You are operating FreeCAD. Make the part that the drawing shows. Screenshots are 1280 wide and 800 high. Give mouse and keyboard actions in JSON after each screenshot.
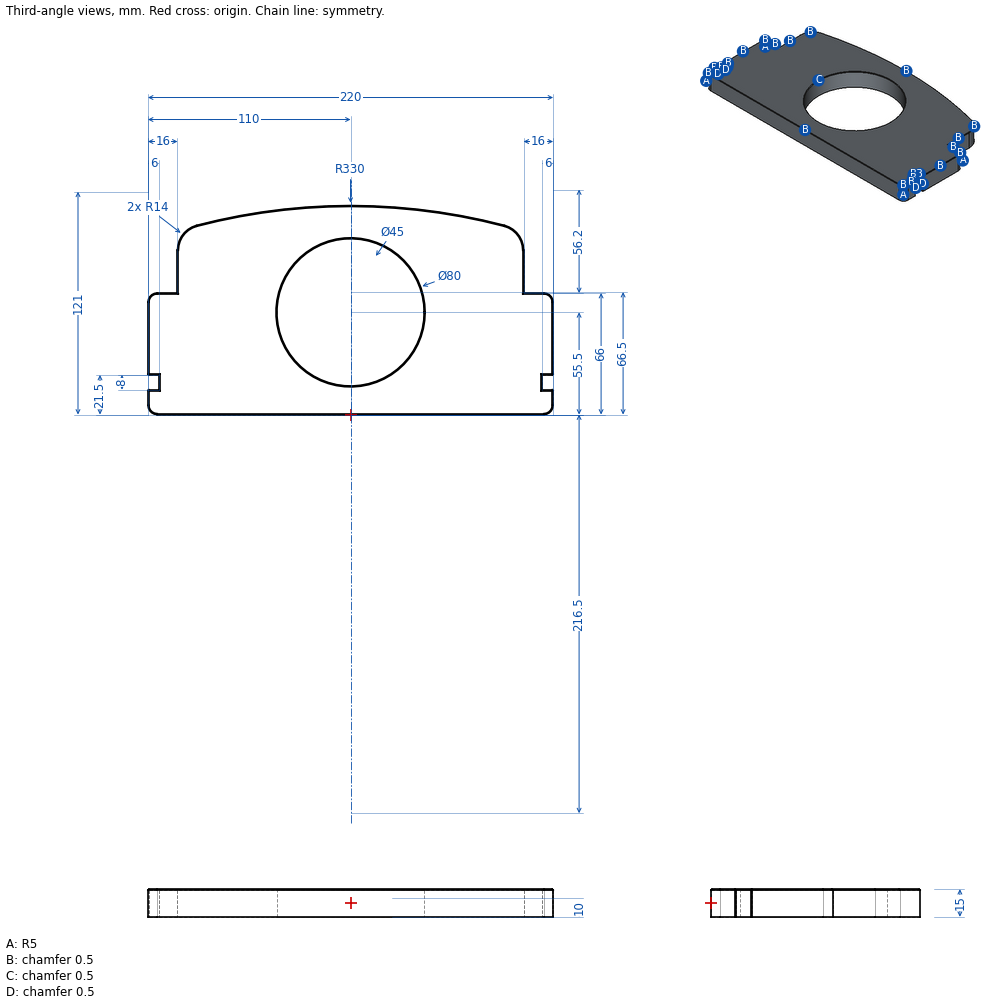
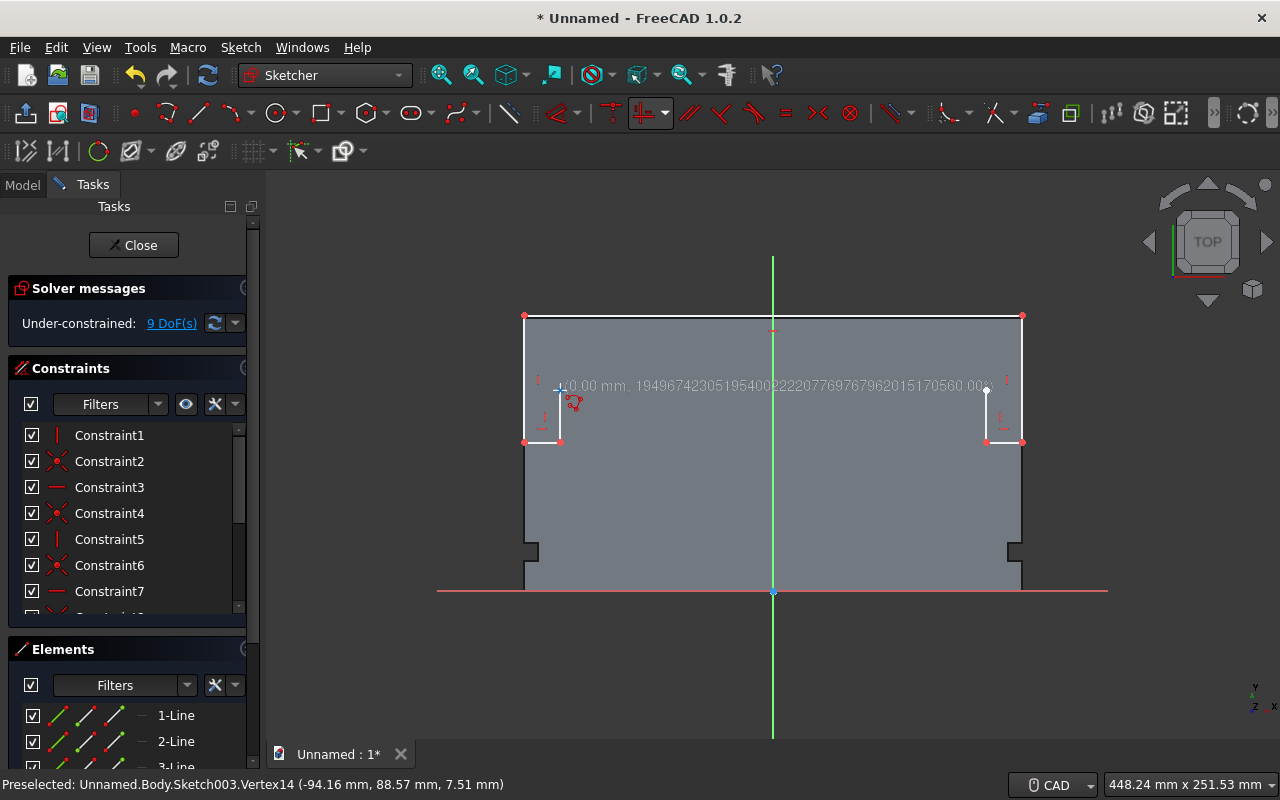
{"action": "left_click", "coordinate": [232, 114]}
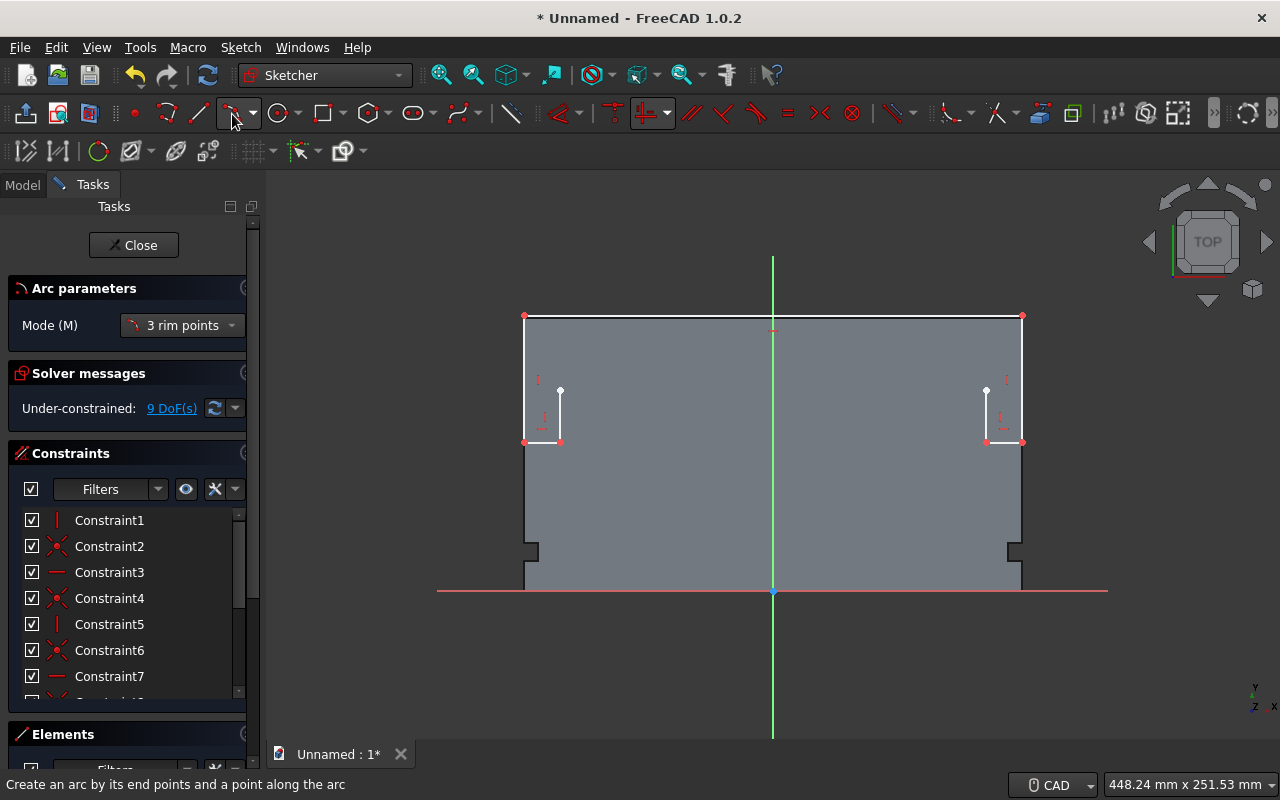
{"action": "left_click", "coordinate": [560, 391]}
{"action": "left_click", "coordinate": [584, 359]}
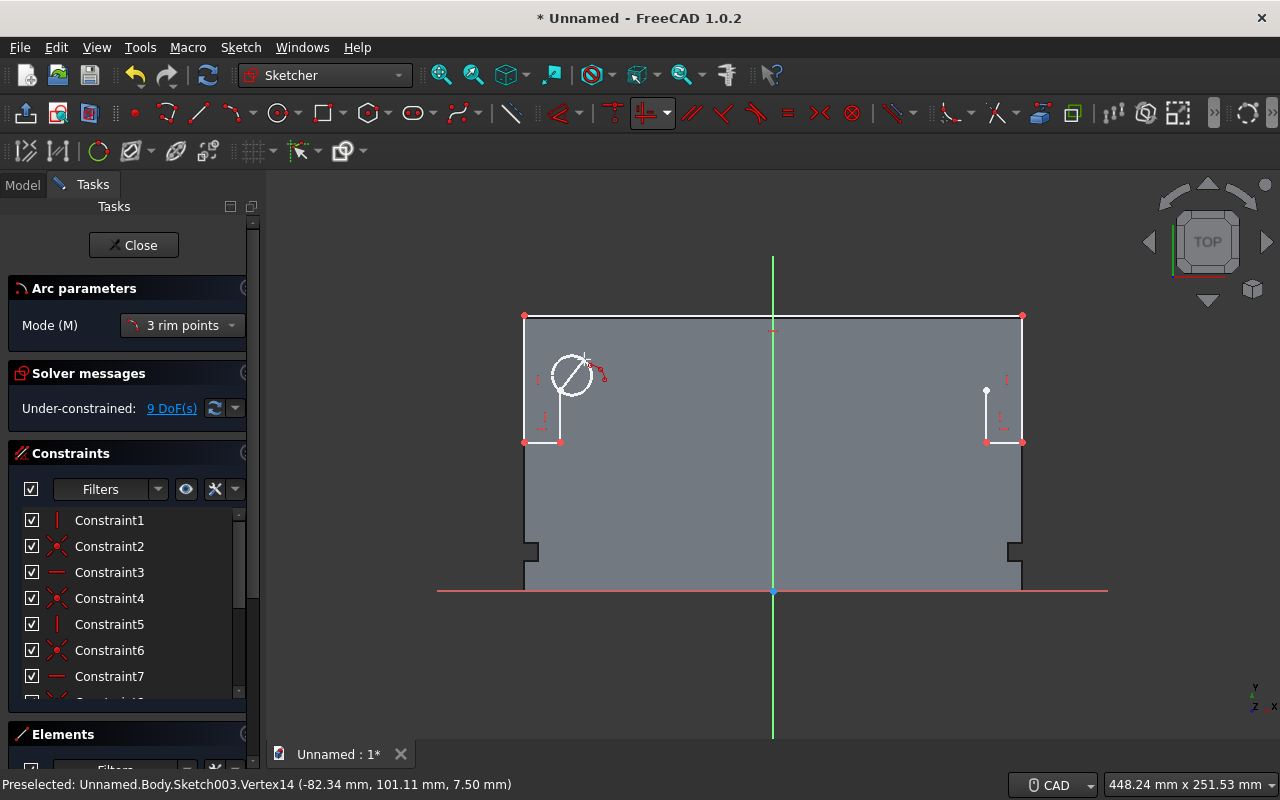
{"action": "scroll", "coordinate": [567, 370], "scroll_direction": "up", "scroll_amount": 5}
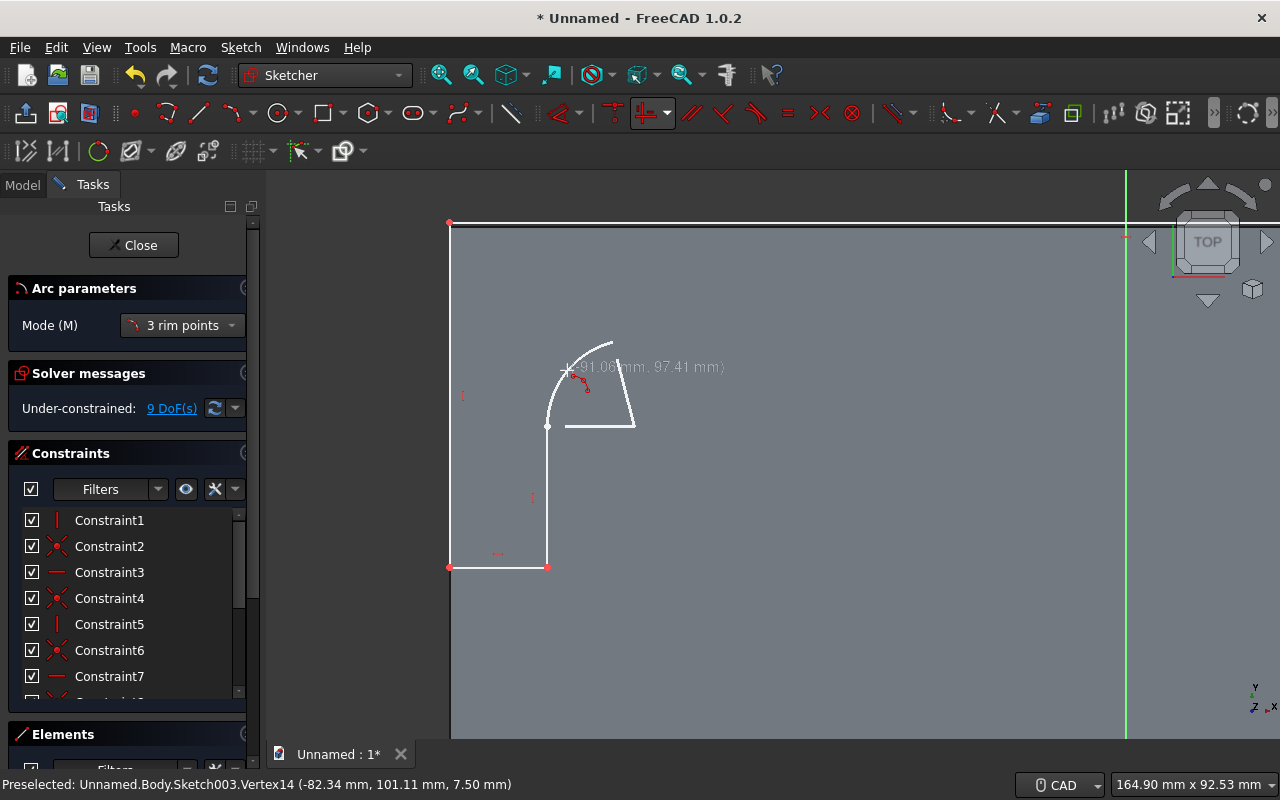
{"action": "left_click", "coordinate": [566, 370]}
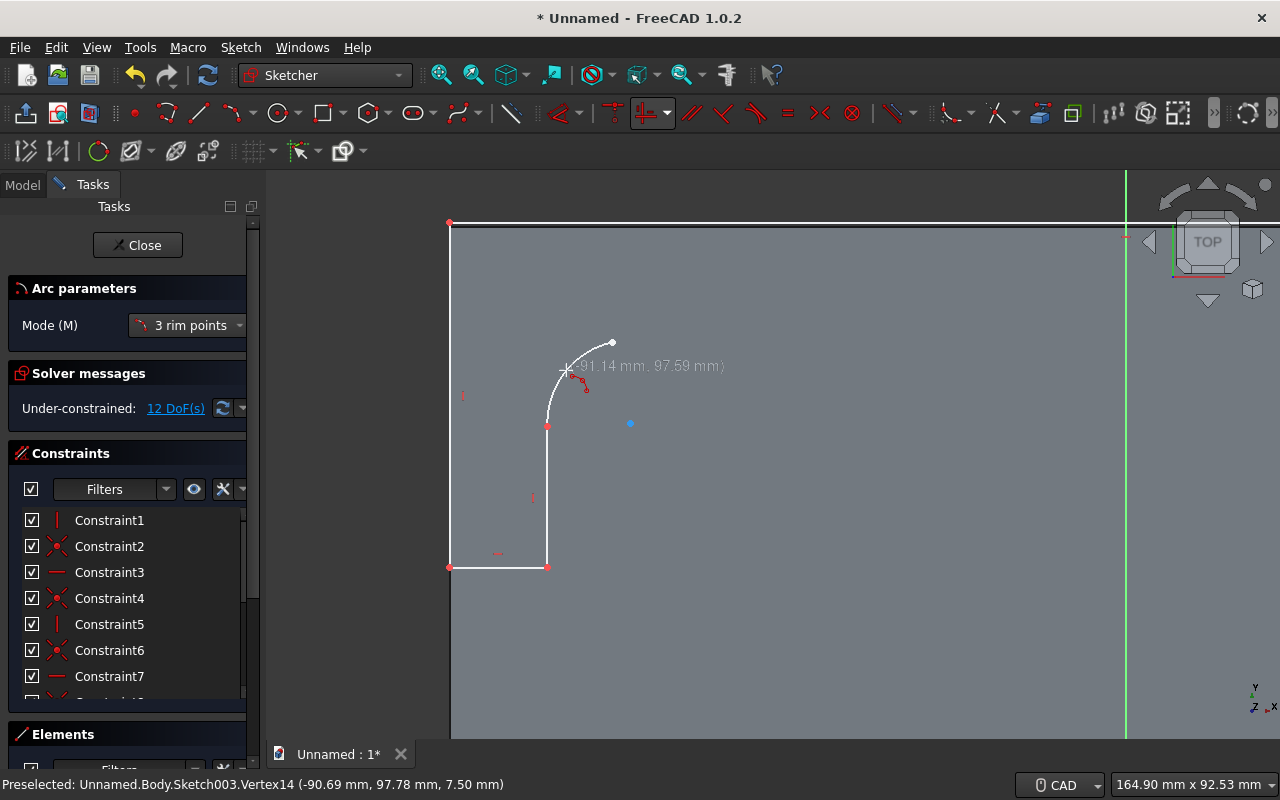
{"action": "left_click", "coordinate": [613, 342]}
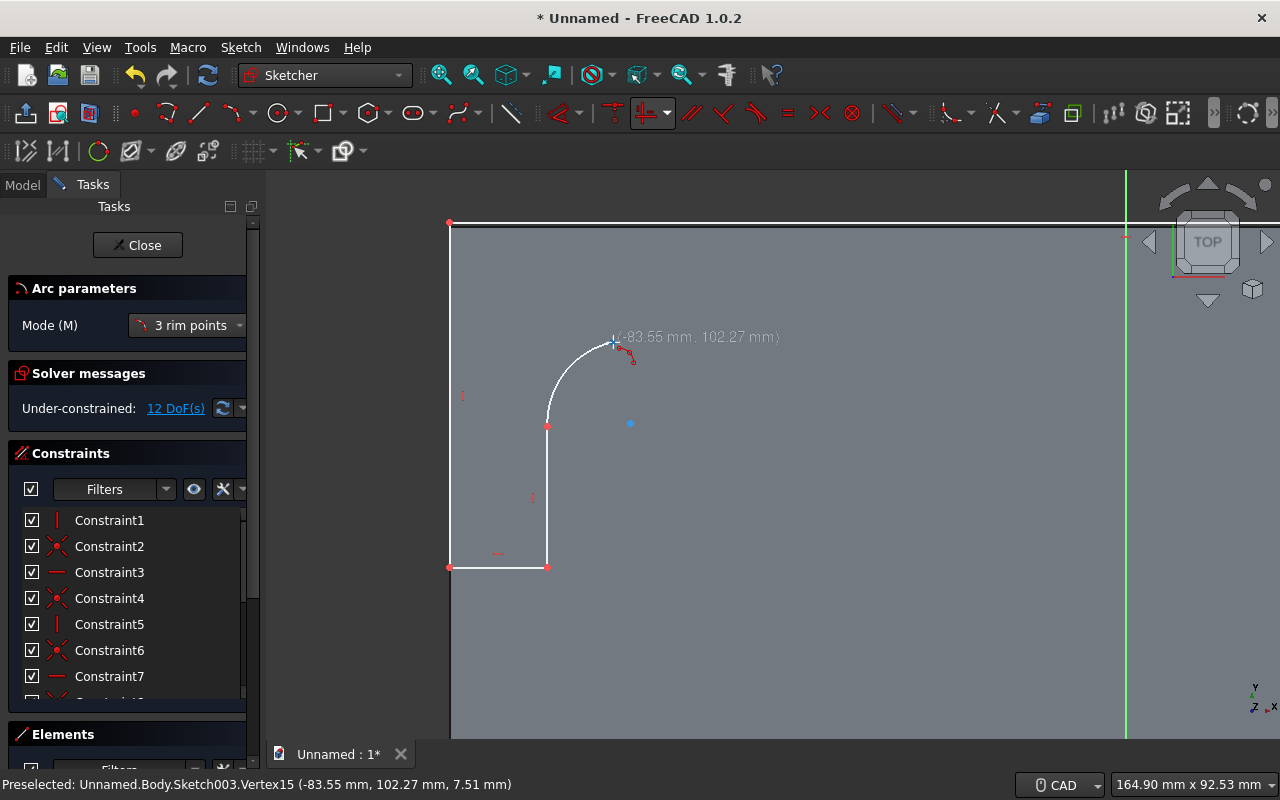
{"action": "scroll", "coordinate": [360, 340], "scroll_direction": "down", "scroll_amount": 4}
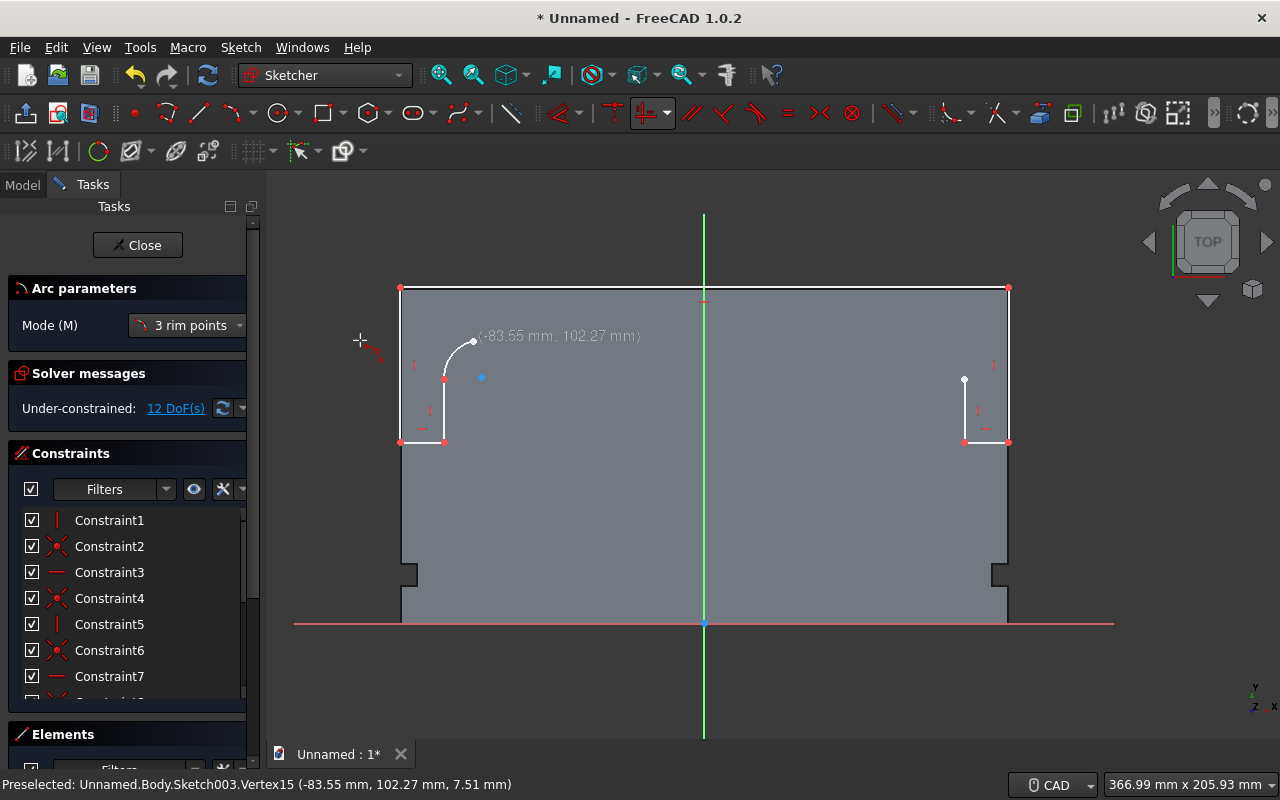
{"action": "left_click", "coordinate": [935, 340]}
{"action": "left_click", "coordinate": [751, 311]}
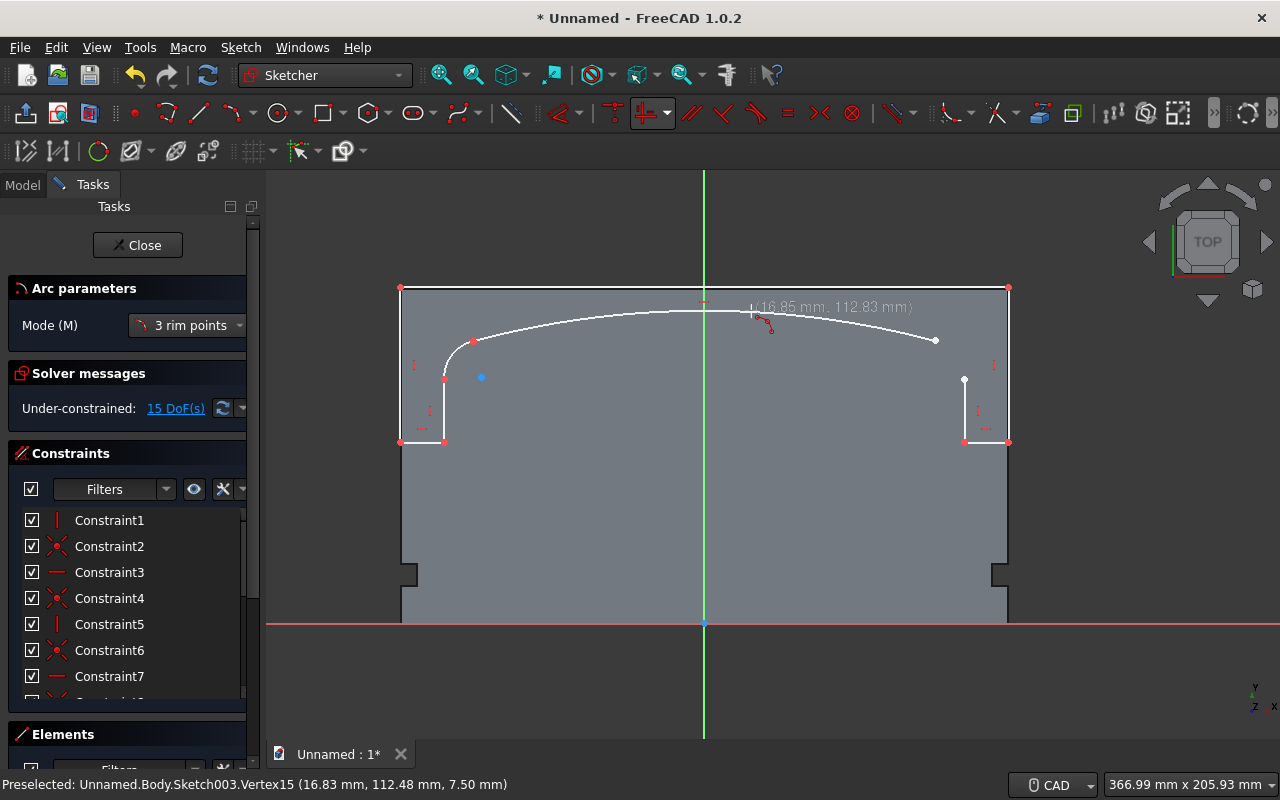
{"action": "left_click", "coordinate": [935, 341]}
{"action": "left_click", "coordinate": [965, 379]}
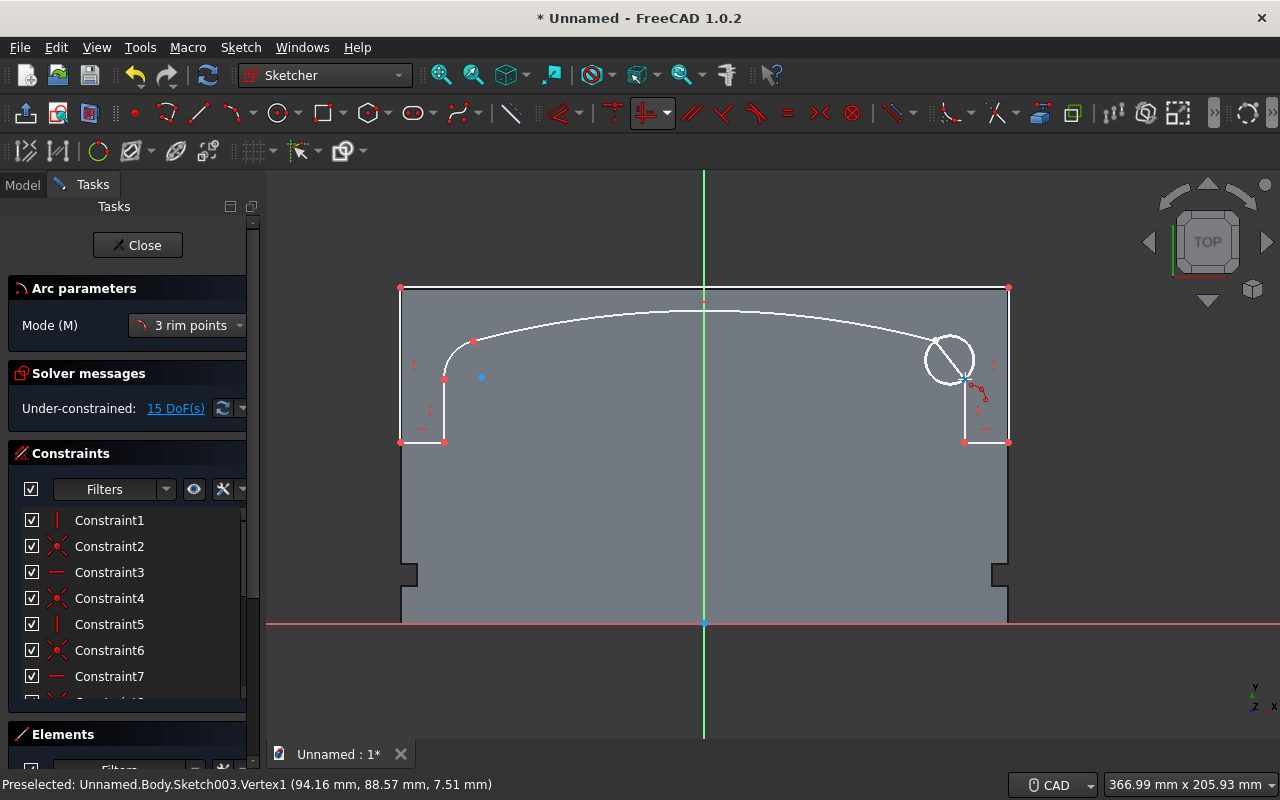
{"action": "scroll", "coordinate": [956, 354], "scroll_direction": "up", "scroll_amount": 4}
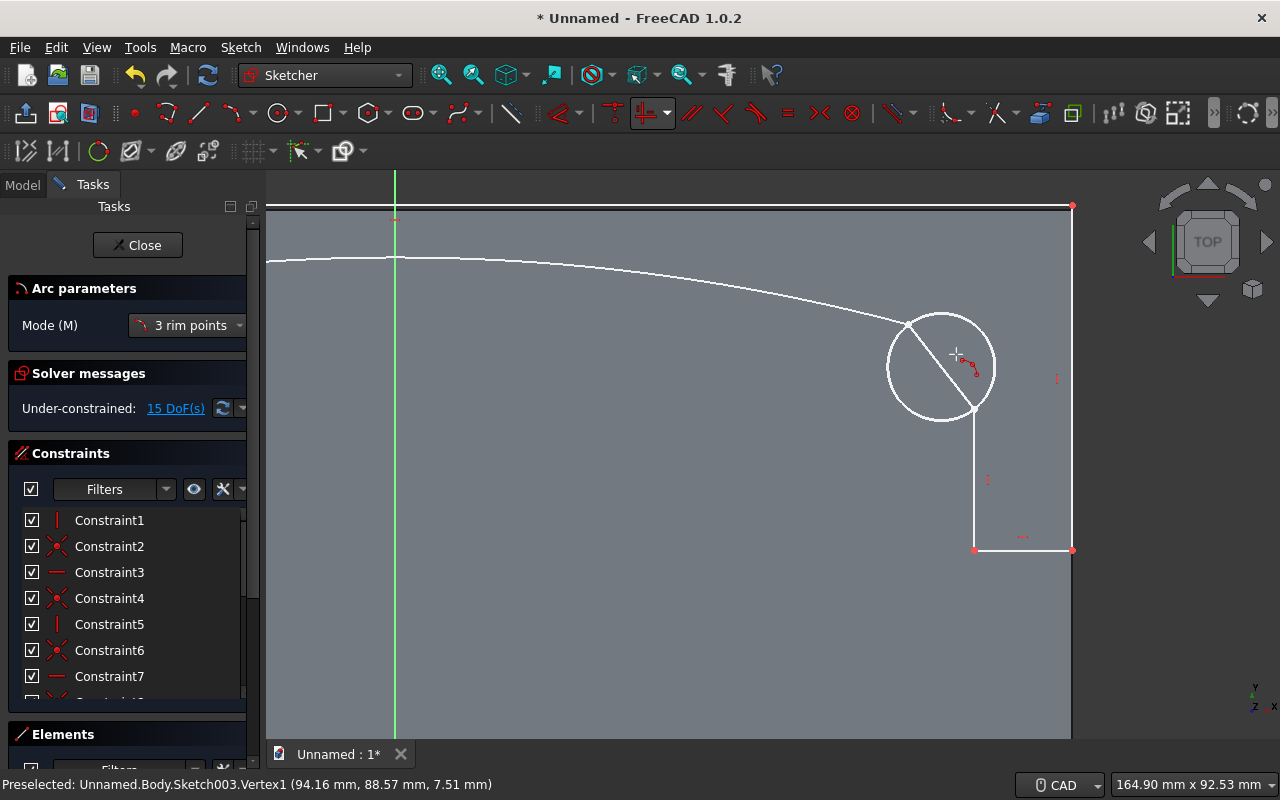
{"action": "left_click", "coordinate": [955, 353]}
{"action": "key", "text": "Escape"}